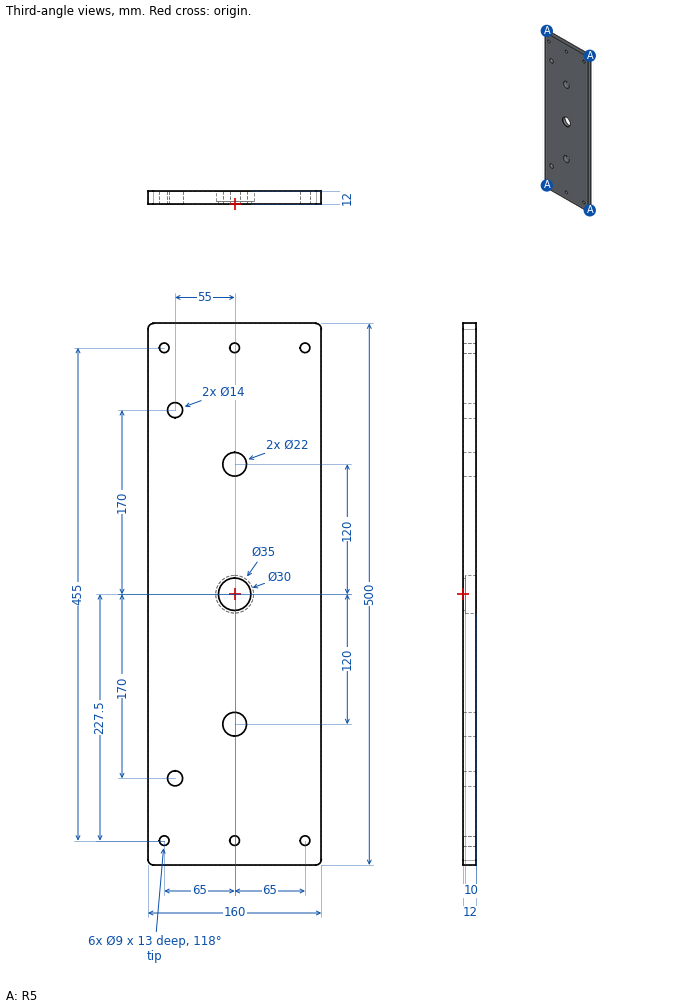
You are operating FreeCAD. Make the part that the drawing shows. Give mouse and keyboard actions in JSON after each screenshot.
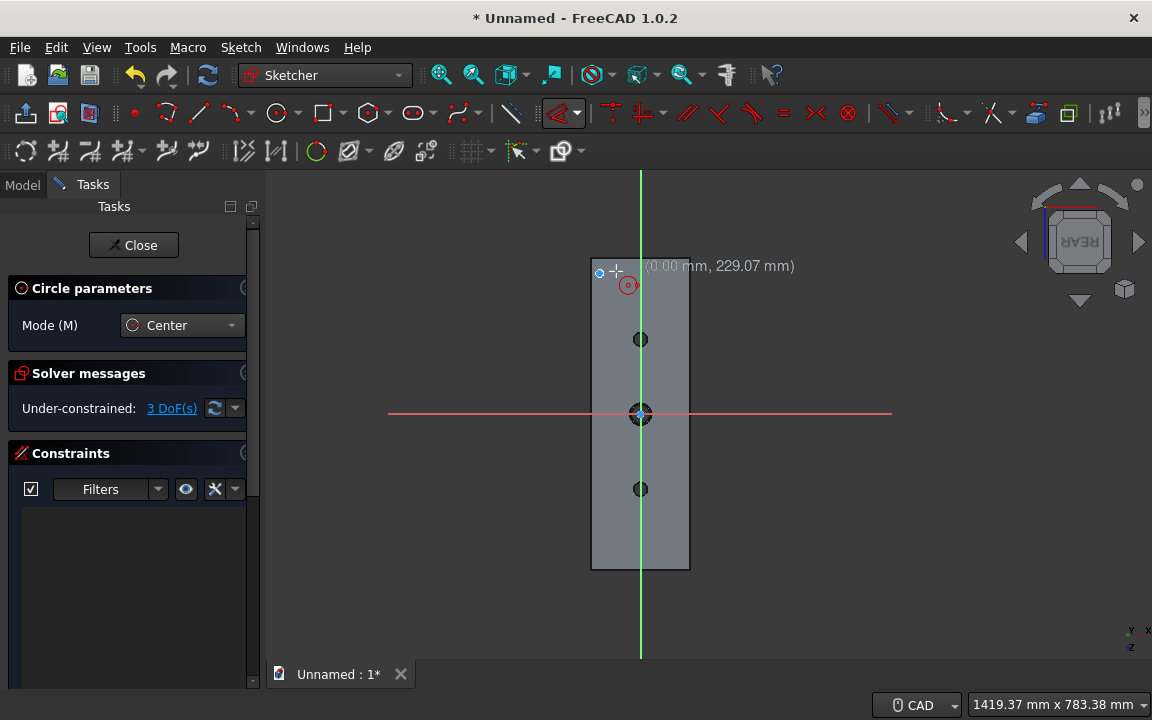
{"action": "left_click", "coordinate": [641, 272]}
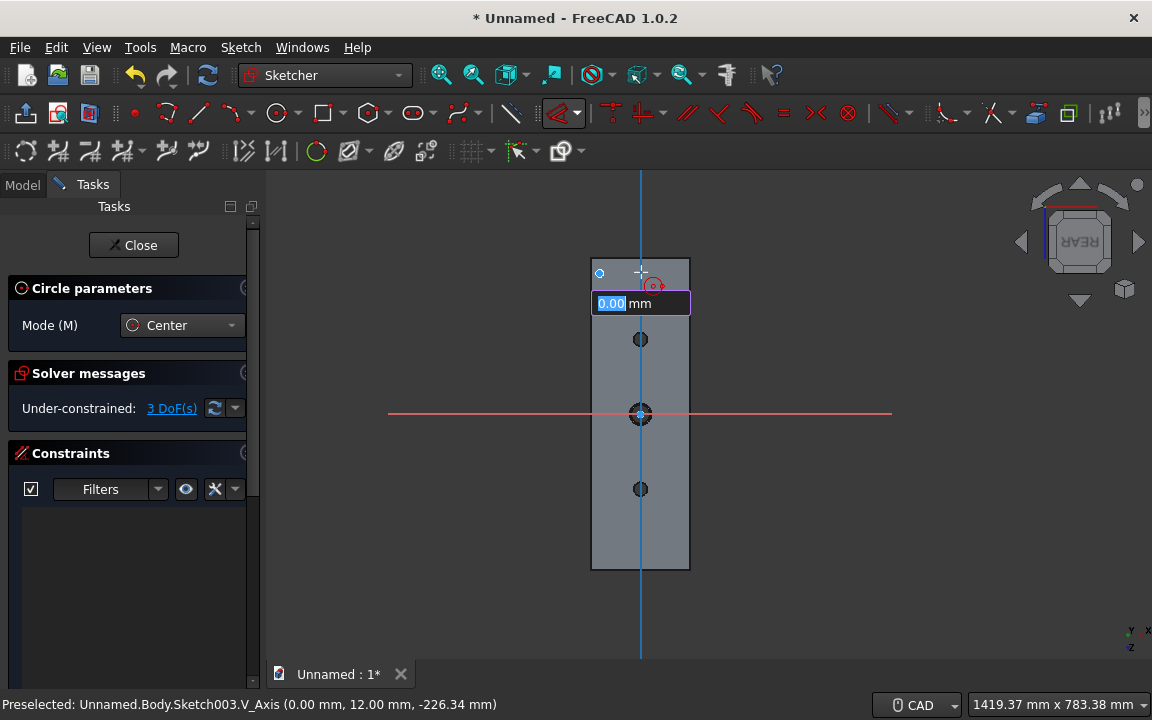
{"action": "scroll", "coordinate": [643, 271], "scroll_direction": "up", "scroll_amount": 9}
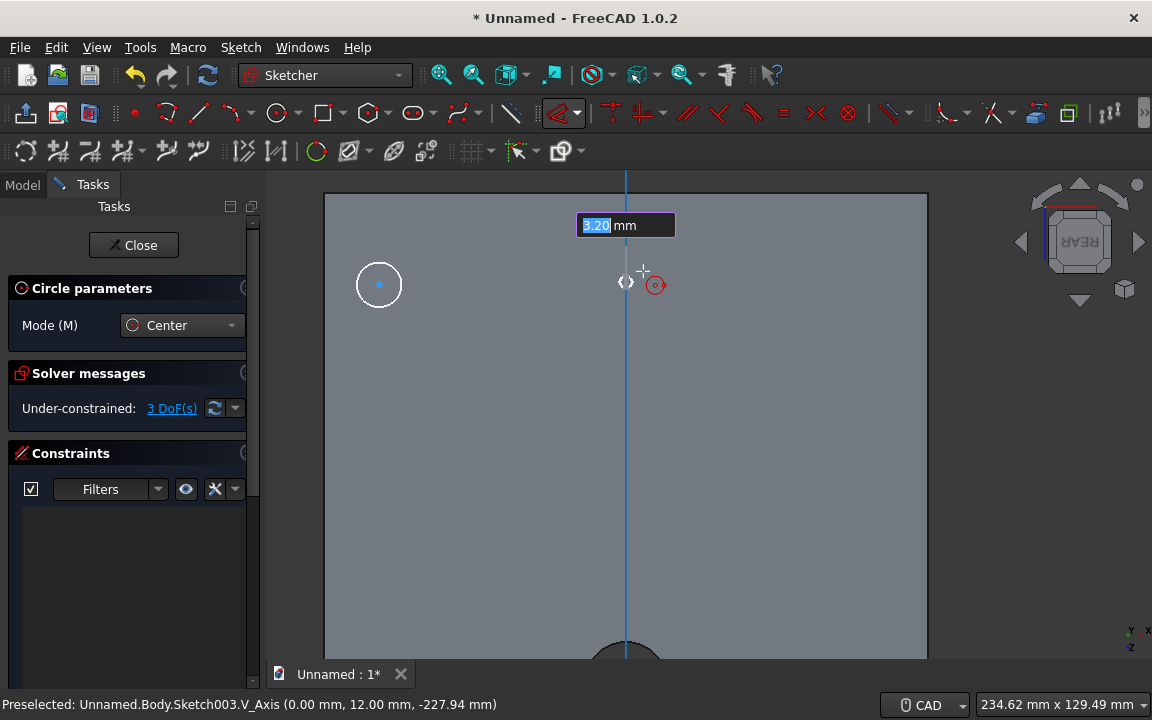
{"action": "left_click", "coordinate": [642, 272]}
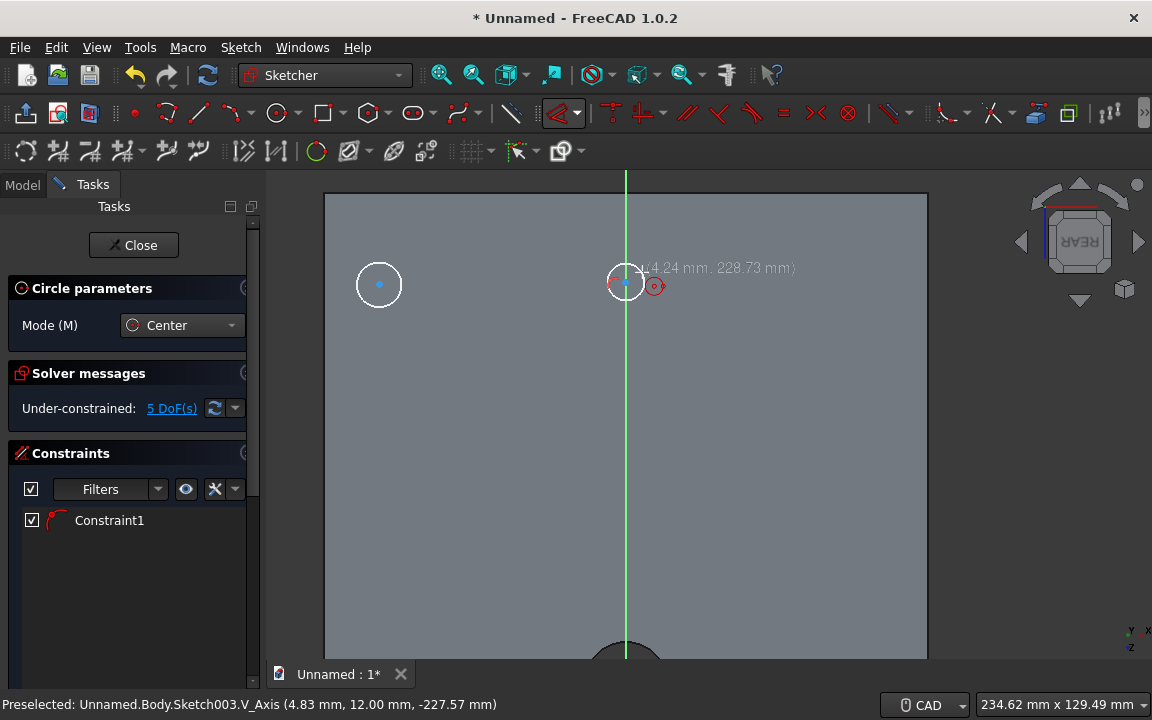
{"action": "scroll", "coordinate": [871, 278], "scroll_direction": "up", "scroll_amount": 2}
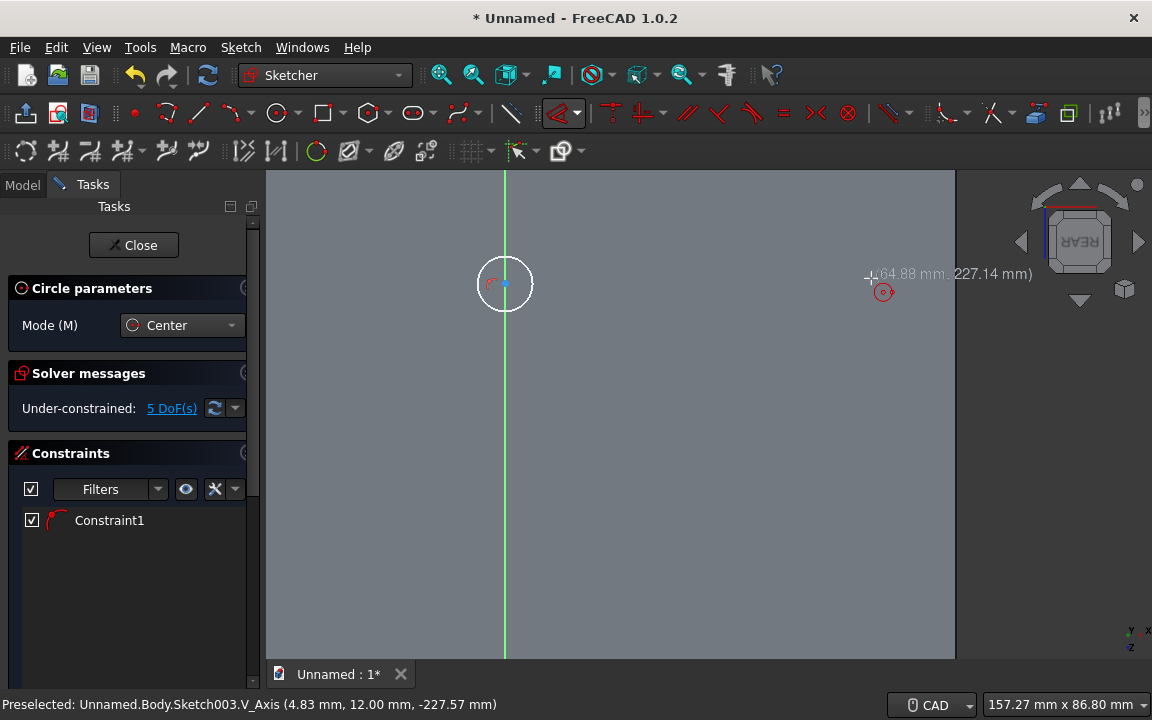
{"action": "scroll", "coordinate": [657, 272], "scroll_direction": "down", "scroll_amount": 11}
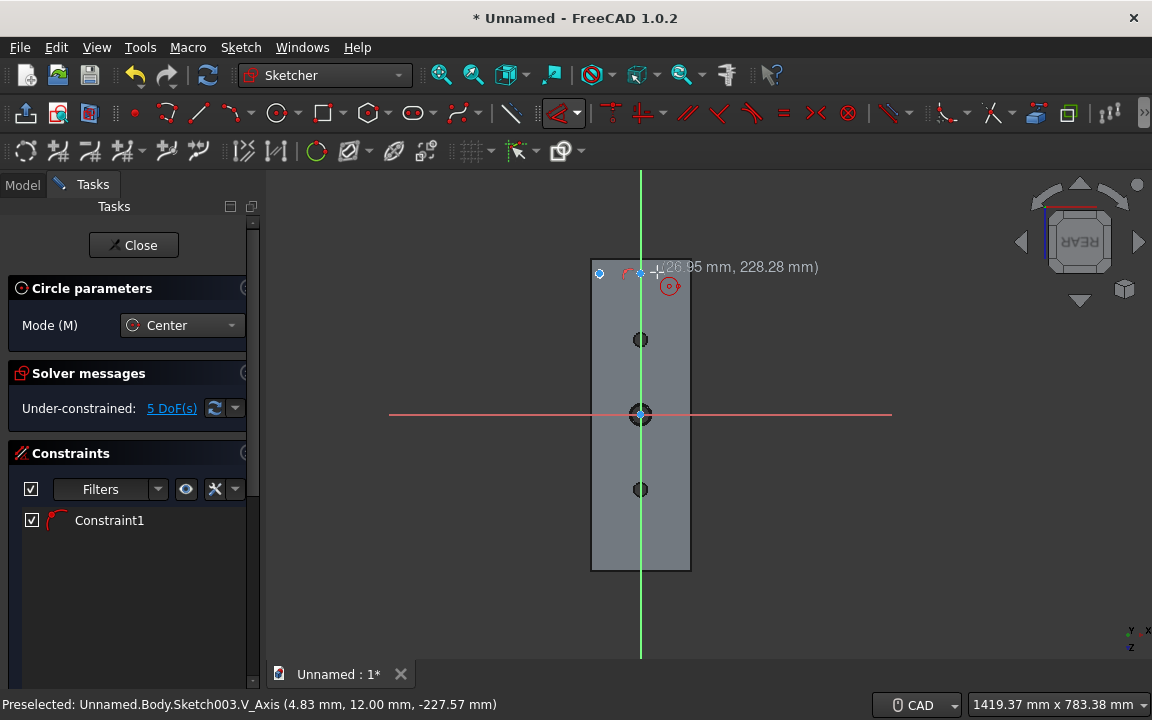
{"action": "left_click", "coordinate": [681, 273]}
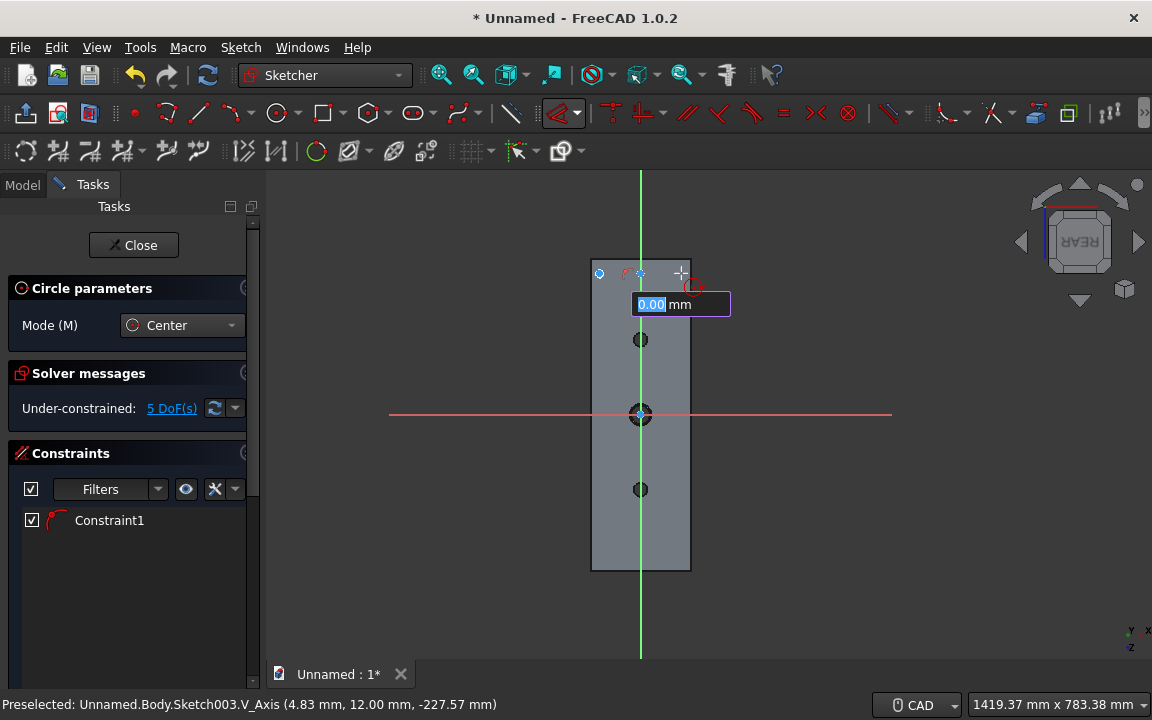
{"action": "scroll", "coordinate": [683, 271], "scroll_direction": "up", "scroll_amount": 9}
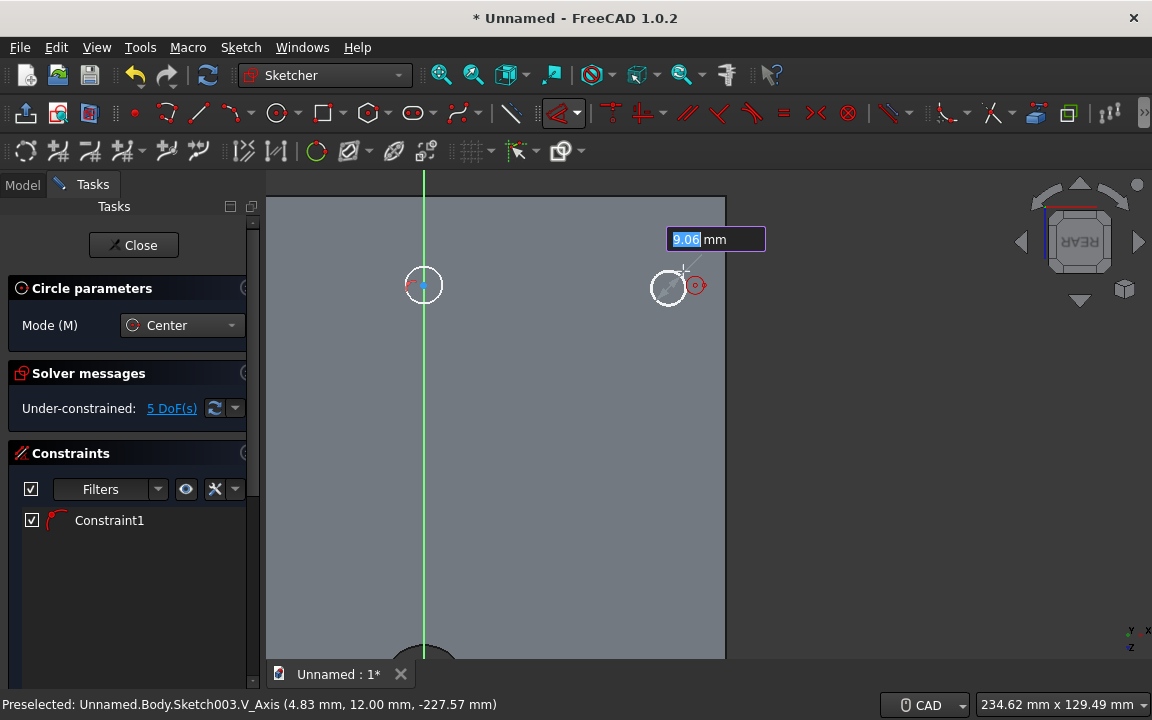
{"action": "left_click", "coordinate": [681, 269]}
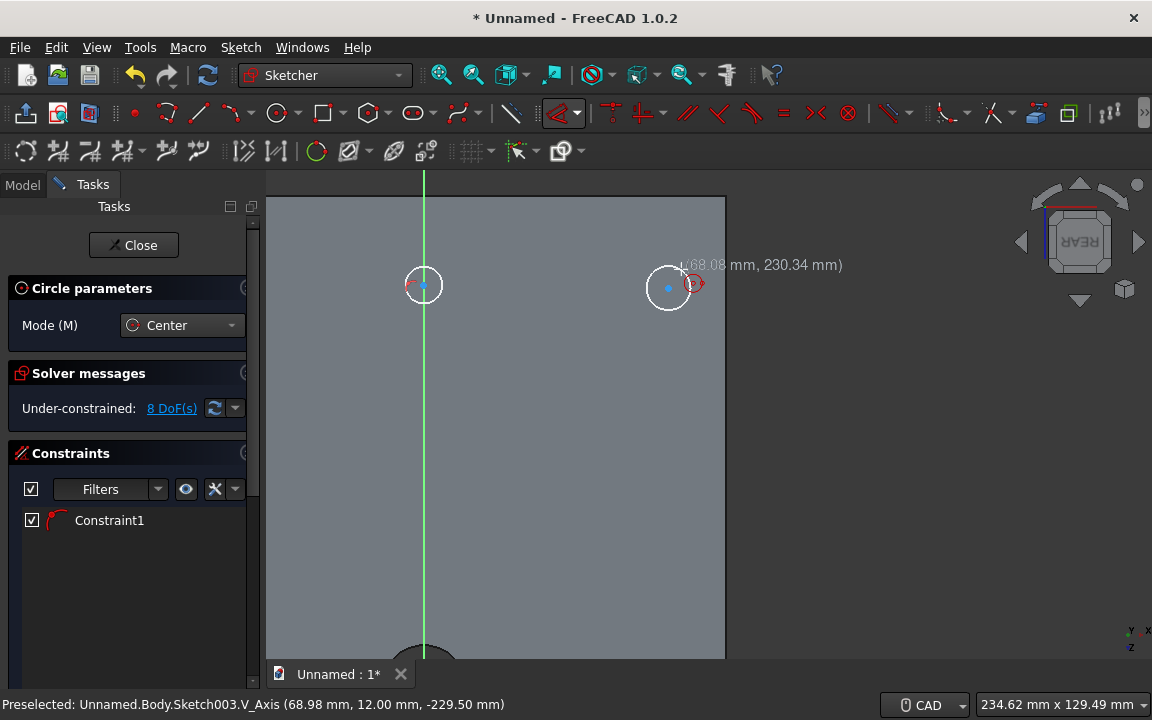
{"action": "scroll", "coordinate": [683, 271], "scroll_direction": "down", "scroll_amount": 9}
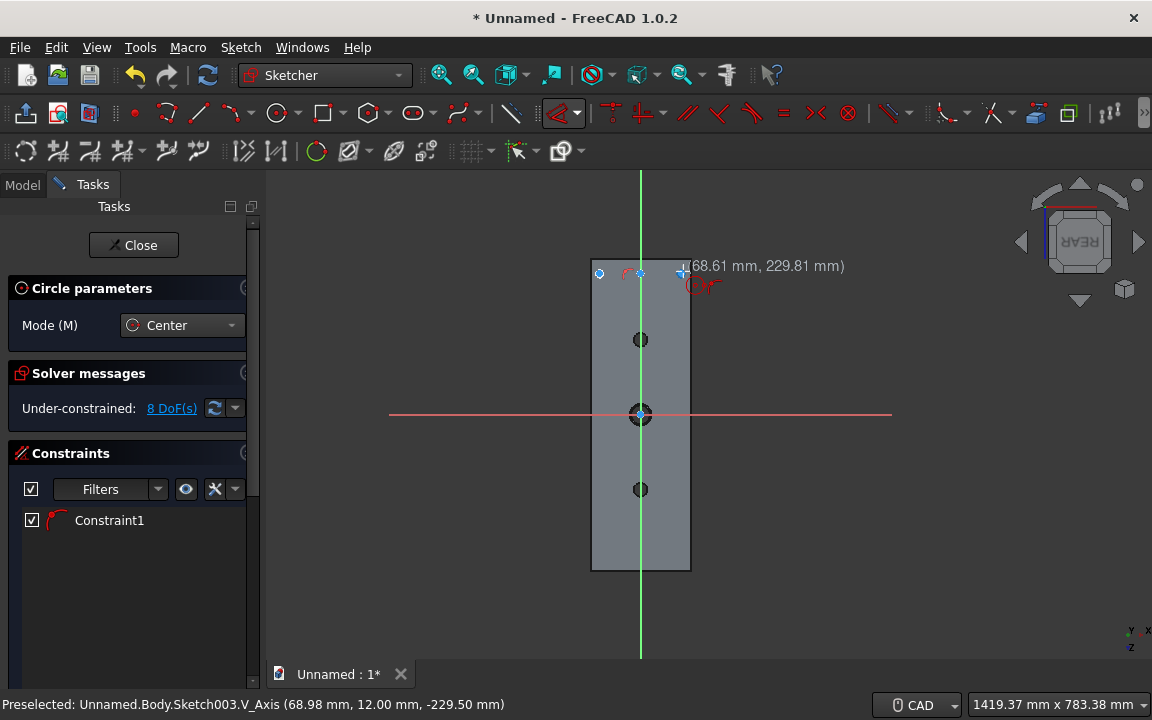
{"action": "scroll", "coordinate": [600, 557], "scroll_direction": "up", "scroll_amount": 11}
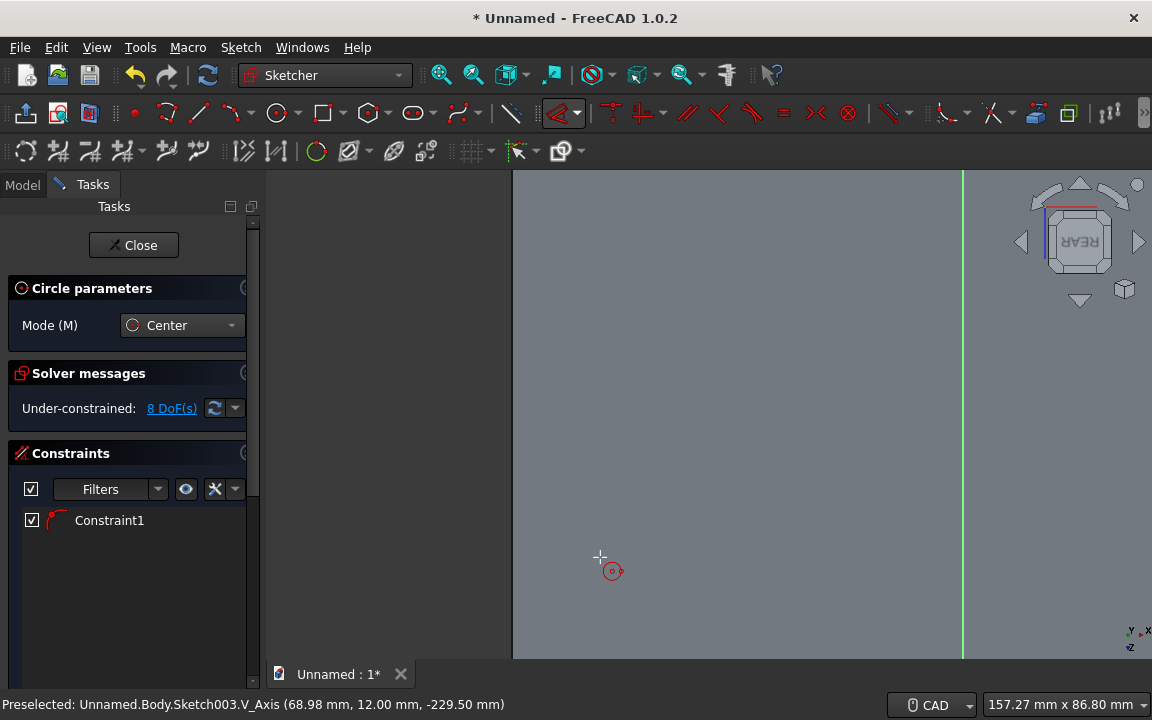
{"action": "scroll", "coordinate": [600, 557], "scroll_direction": "down", "scroll_amount": 11}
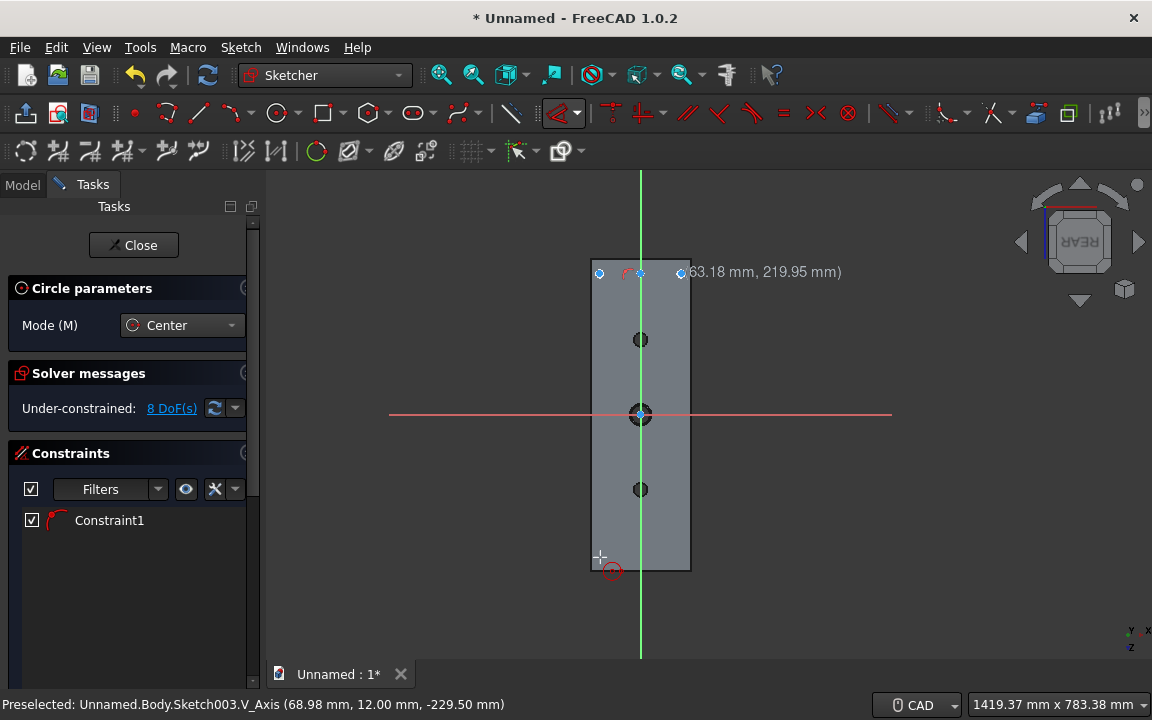
{"action": "left_click", "coordinate": [600, 557]}